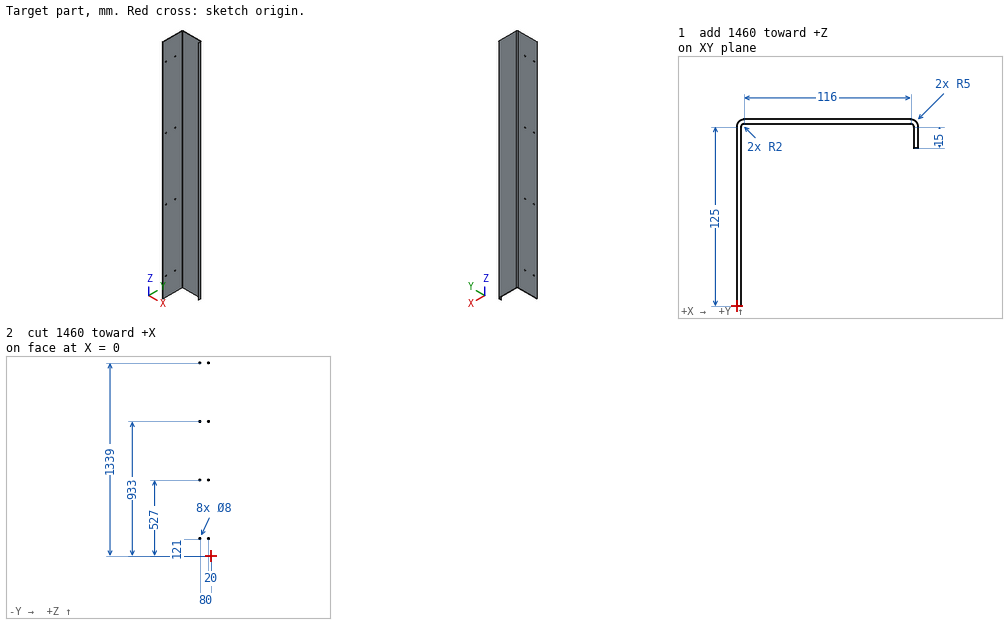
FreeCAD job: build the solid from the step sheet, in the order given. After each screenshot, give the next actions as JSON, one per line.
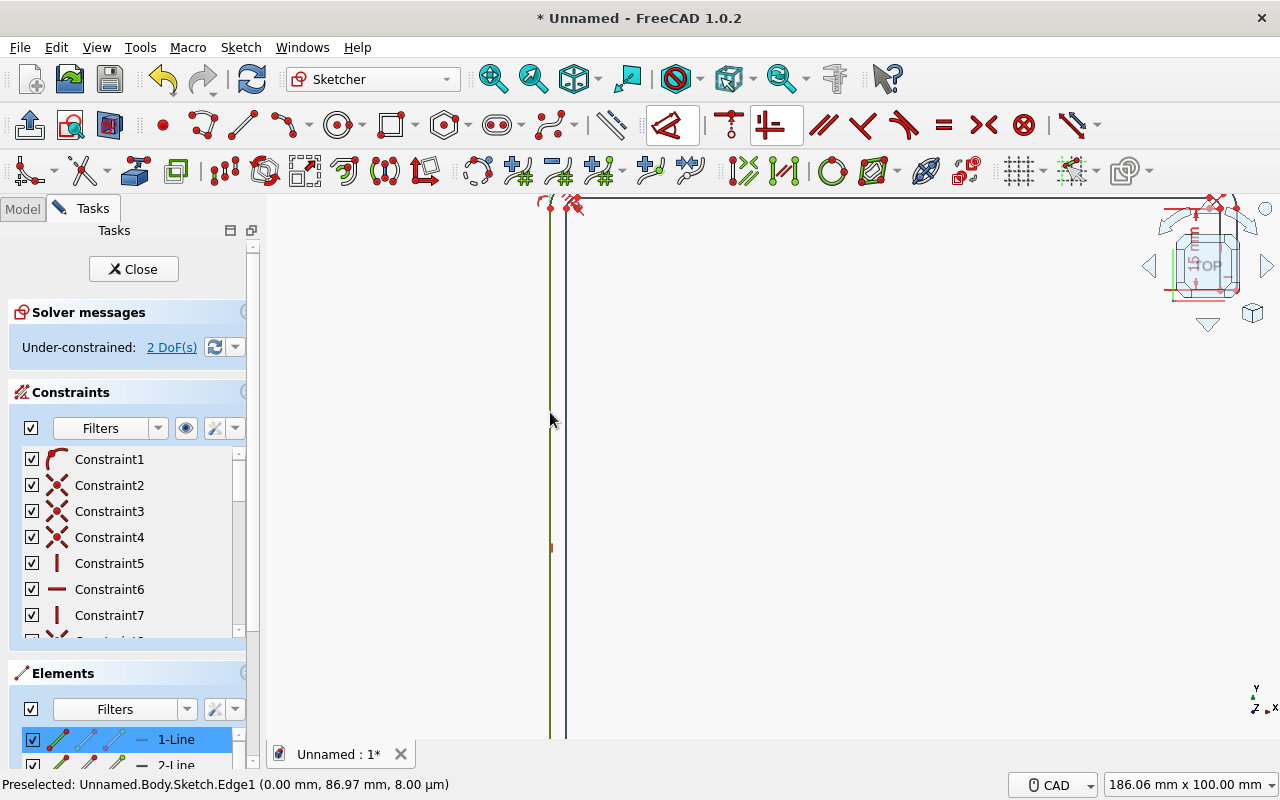
{"action": "left_click", "coordinate": [694, 126]}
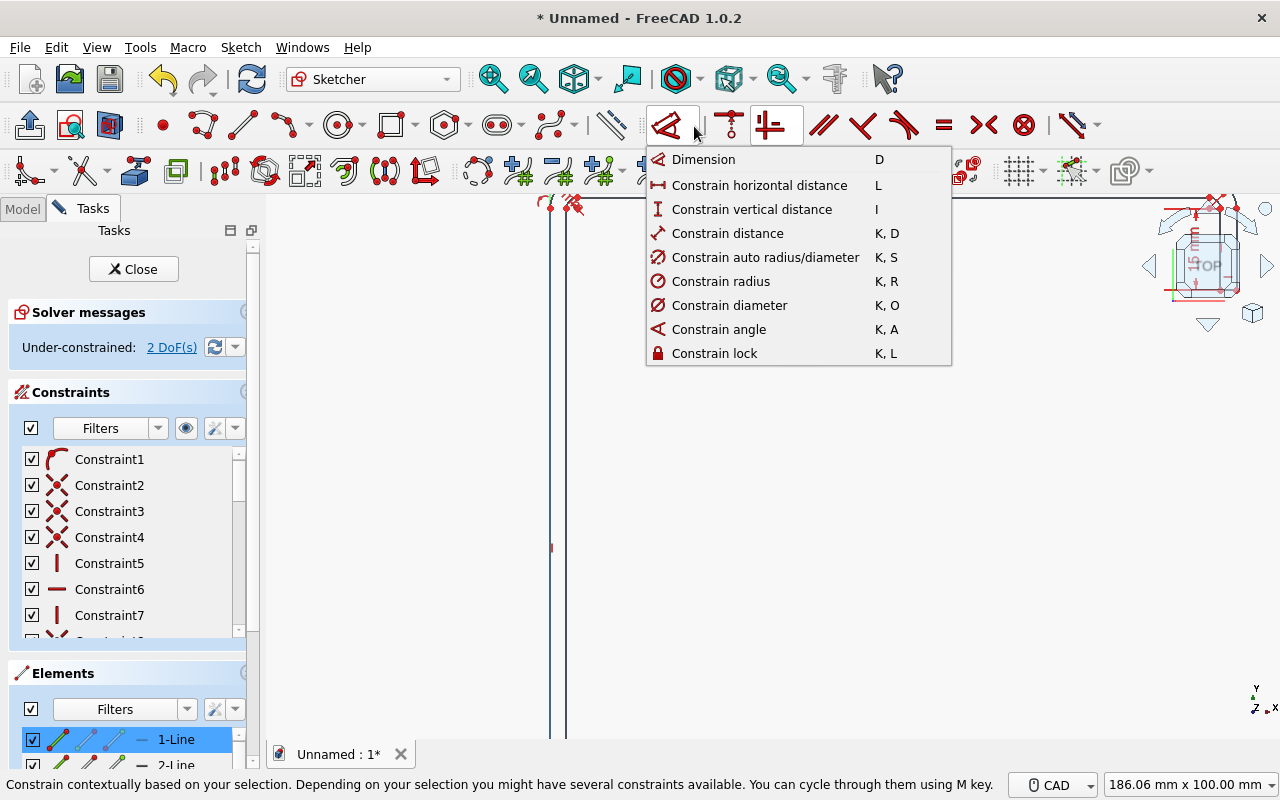
{"action": "left_click", "coordinate": [799, 209]}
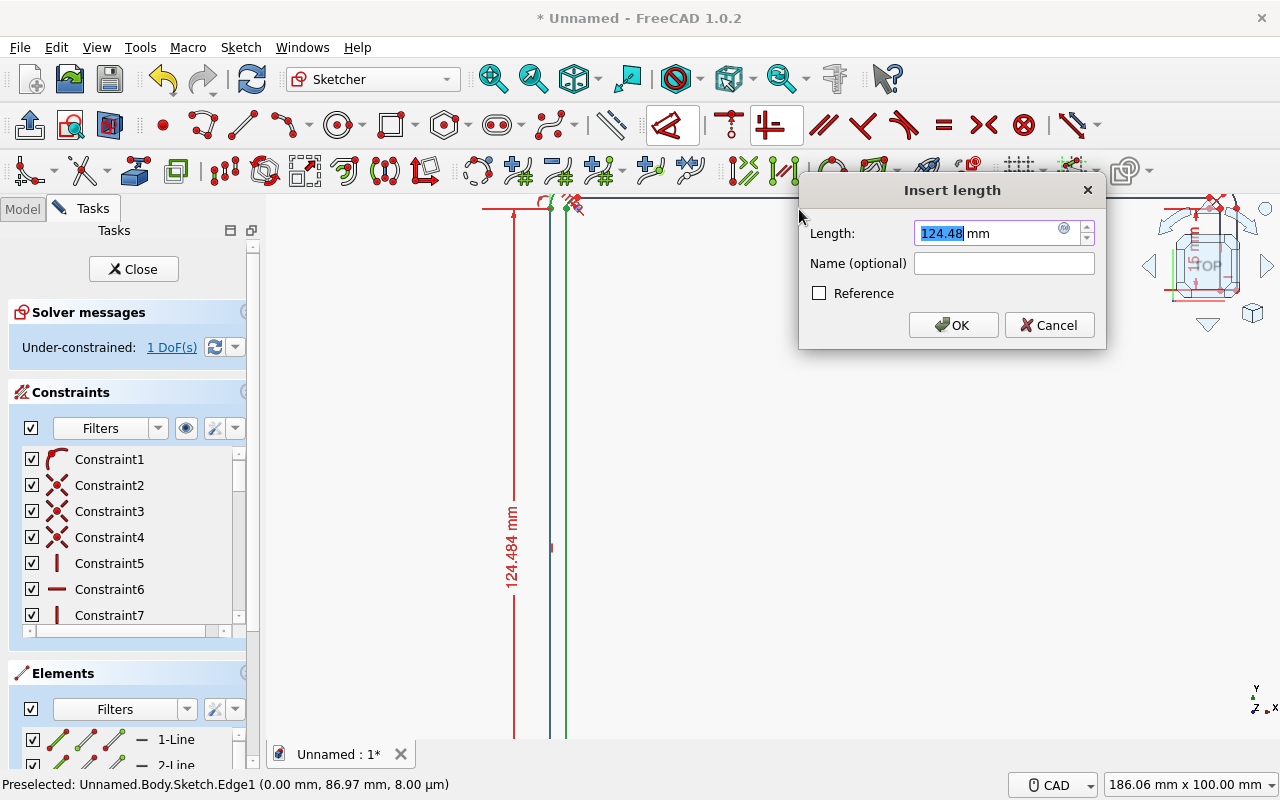
{"action": "type", "text": "125"}
{"action": "key", "text": "Return"}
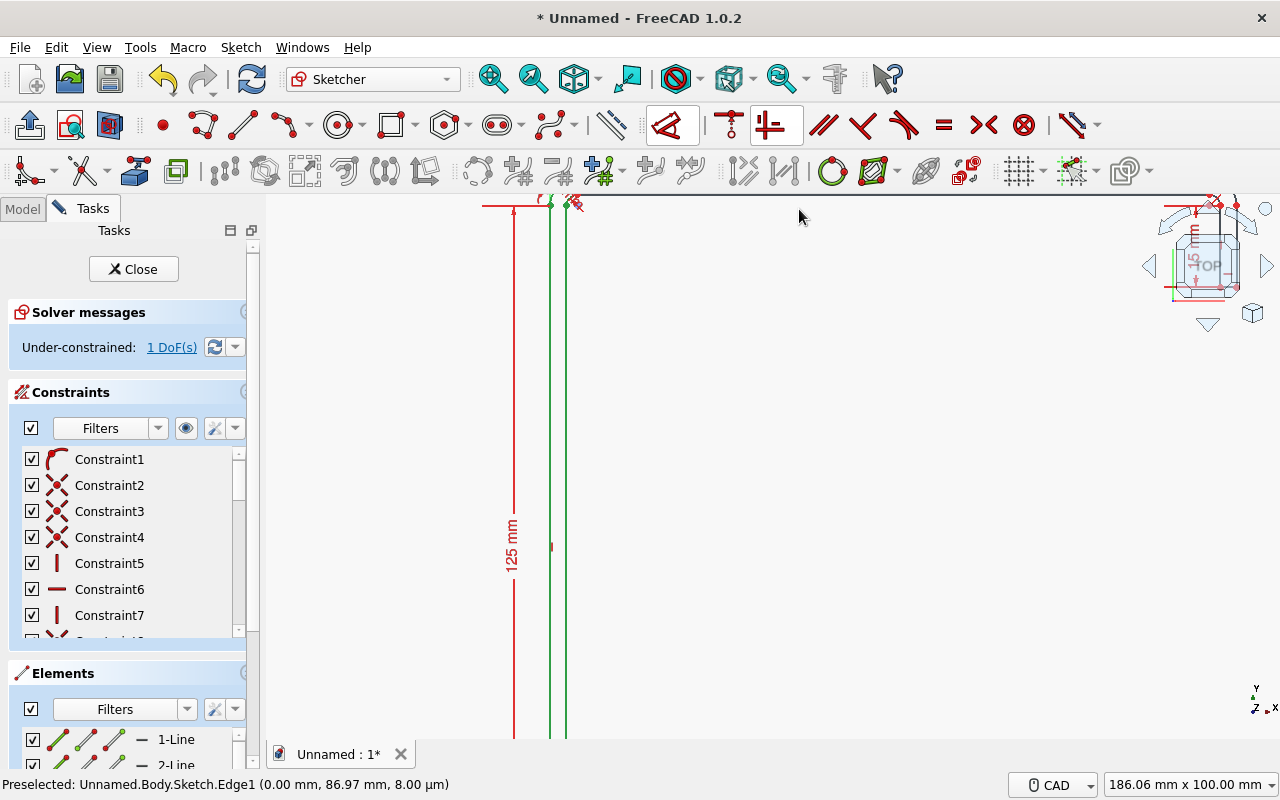
{"action": "scroll", "coordinate": [550, 412], "scroll_direction": "down", "scroll_amount": 4}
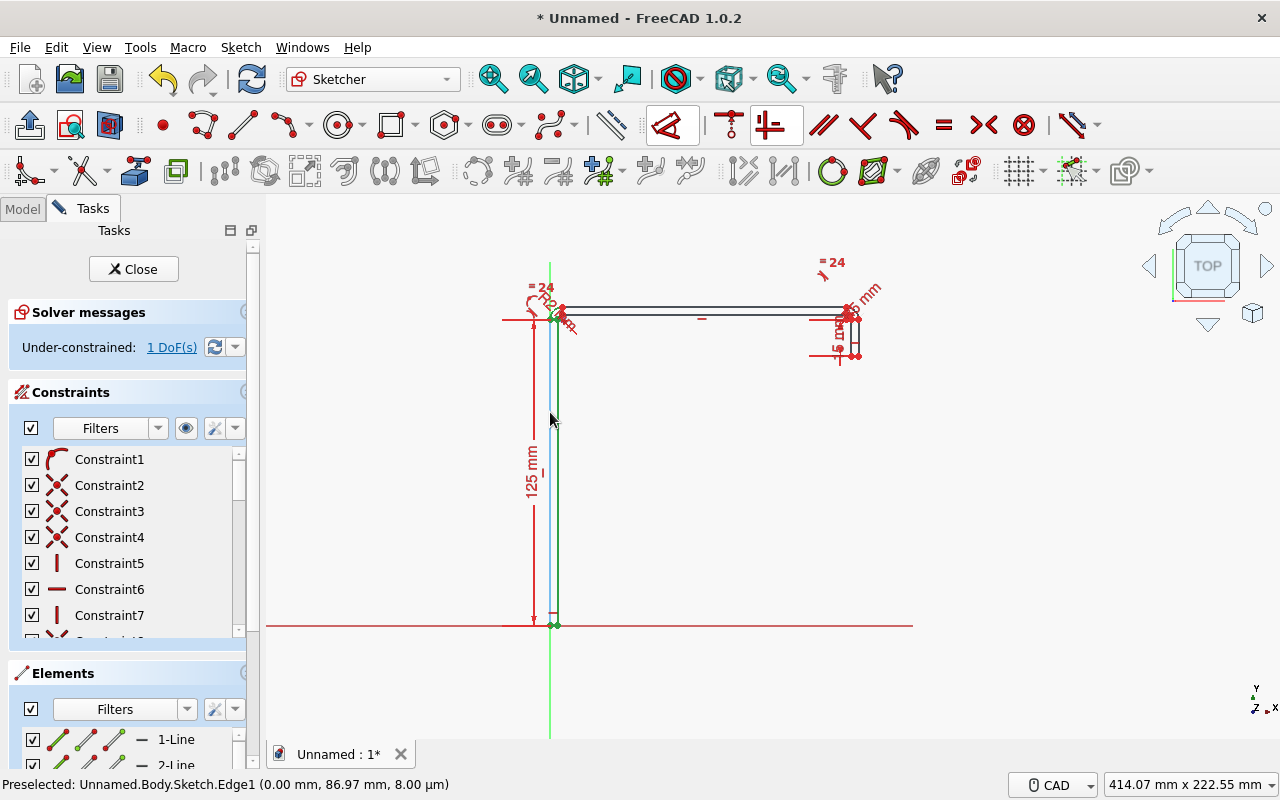
{"action": "scroll", "coordinate": [648, 315], "scroll_direction": "up", "scroll_amount": 4}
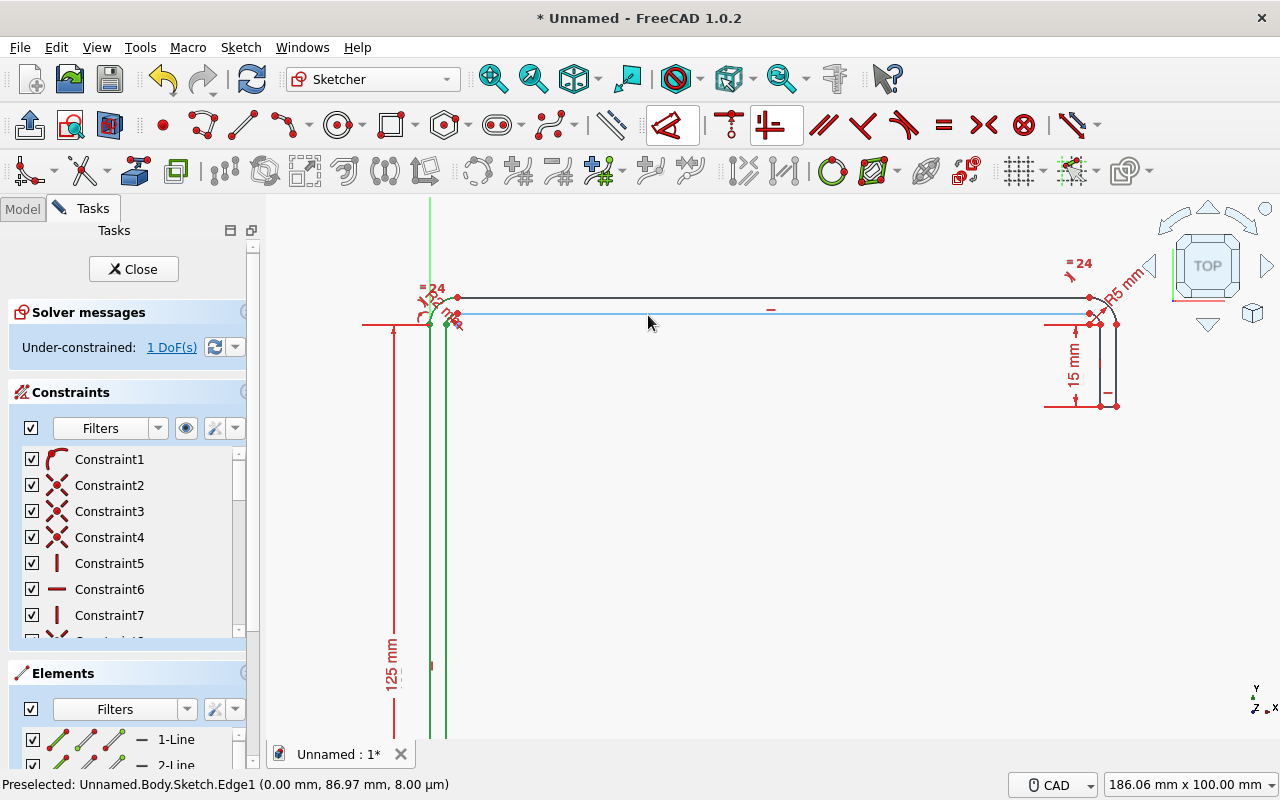
{"action": "left_click", "coordinate": [647, 314]}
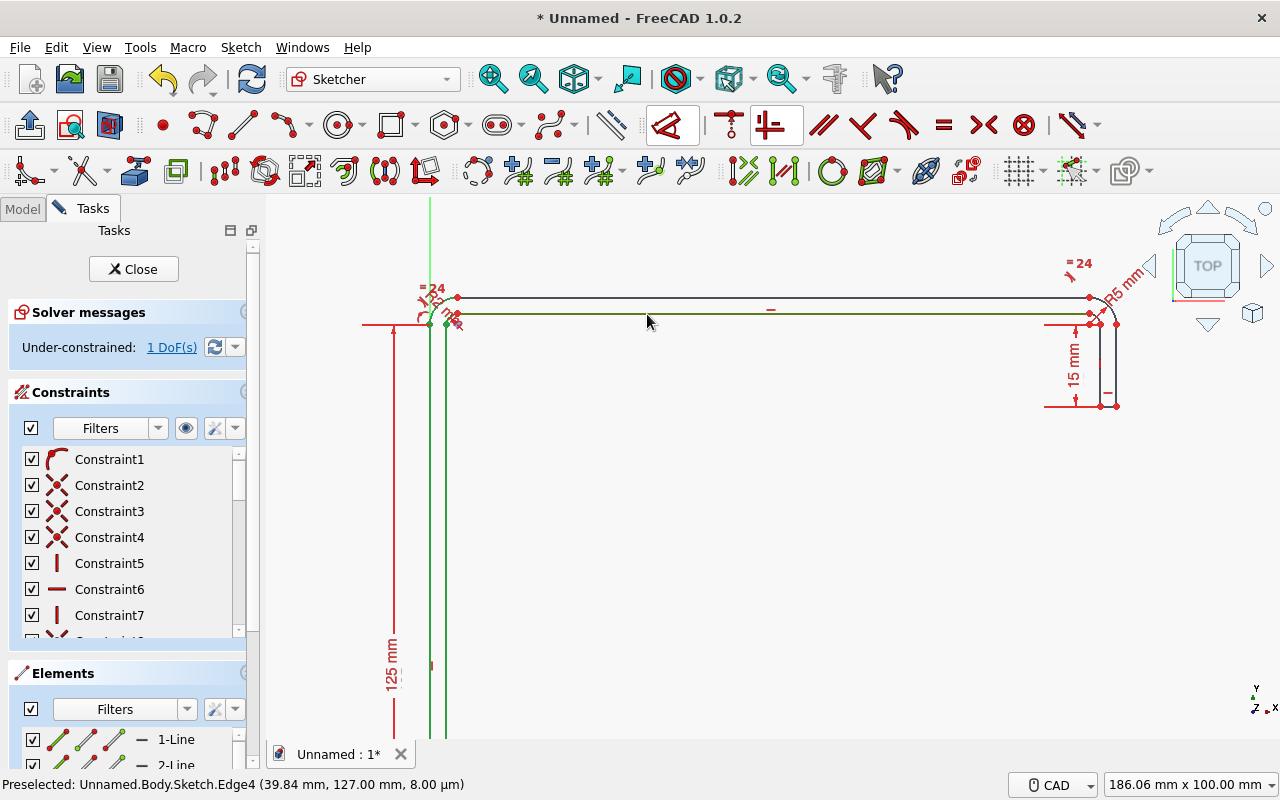
{"action": "key", "text": "l"}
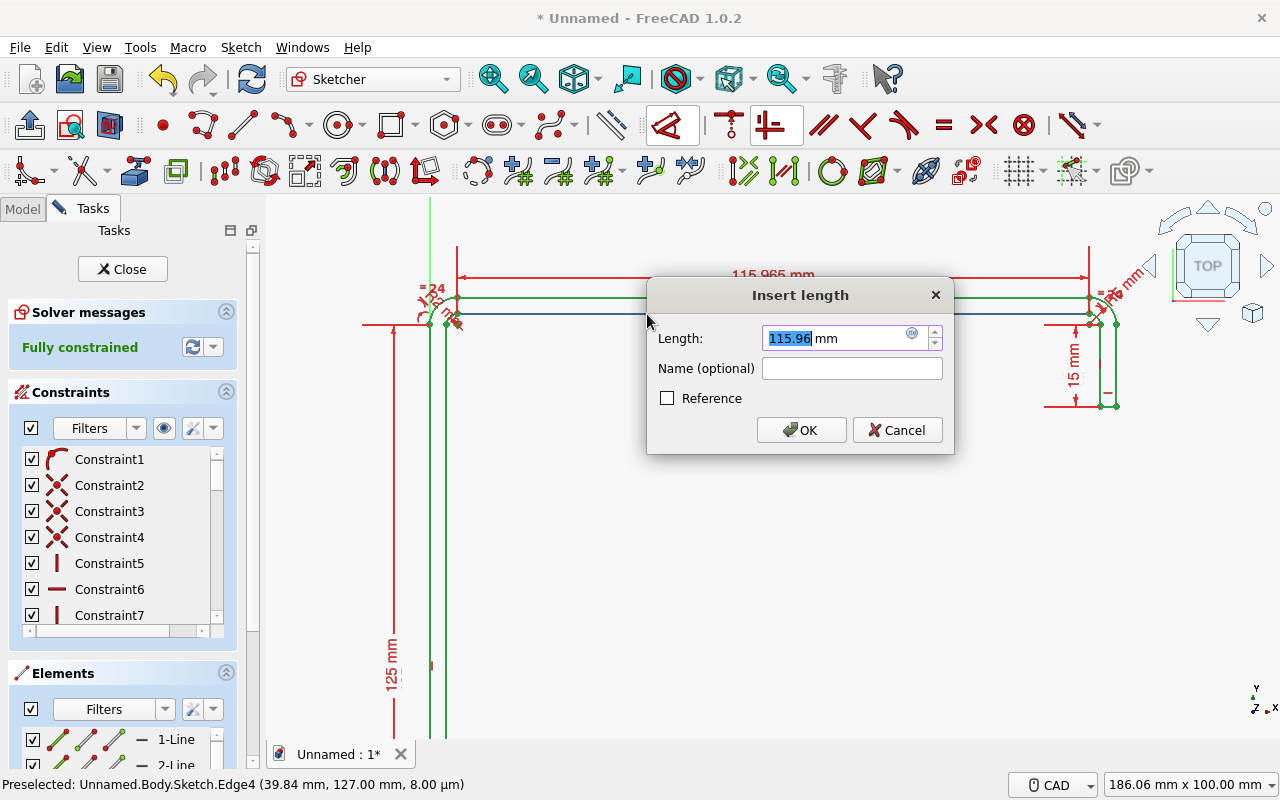
{"action": "type", "text": "116"}
{"action": "key", "text": "Return"}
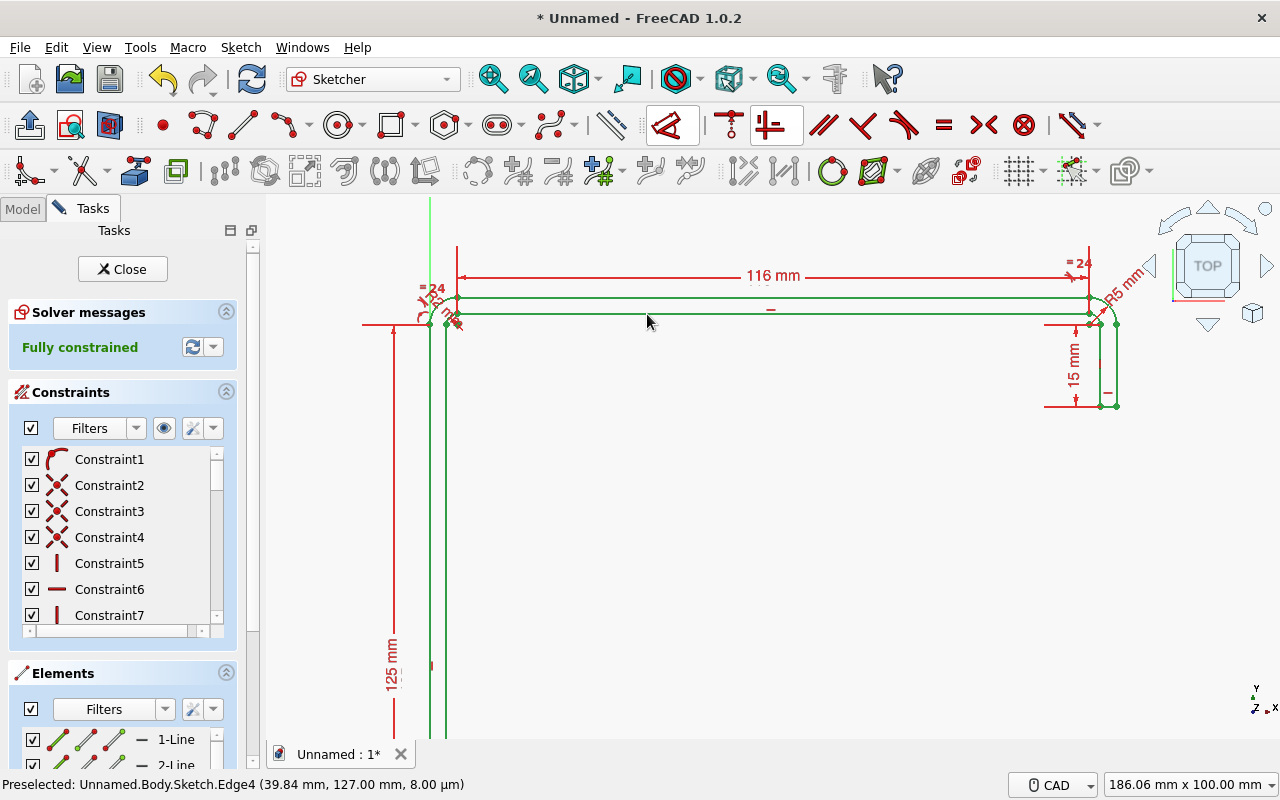
{"action": "left_click", "coordinate": [123, 269]}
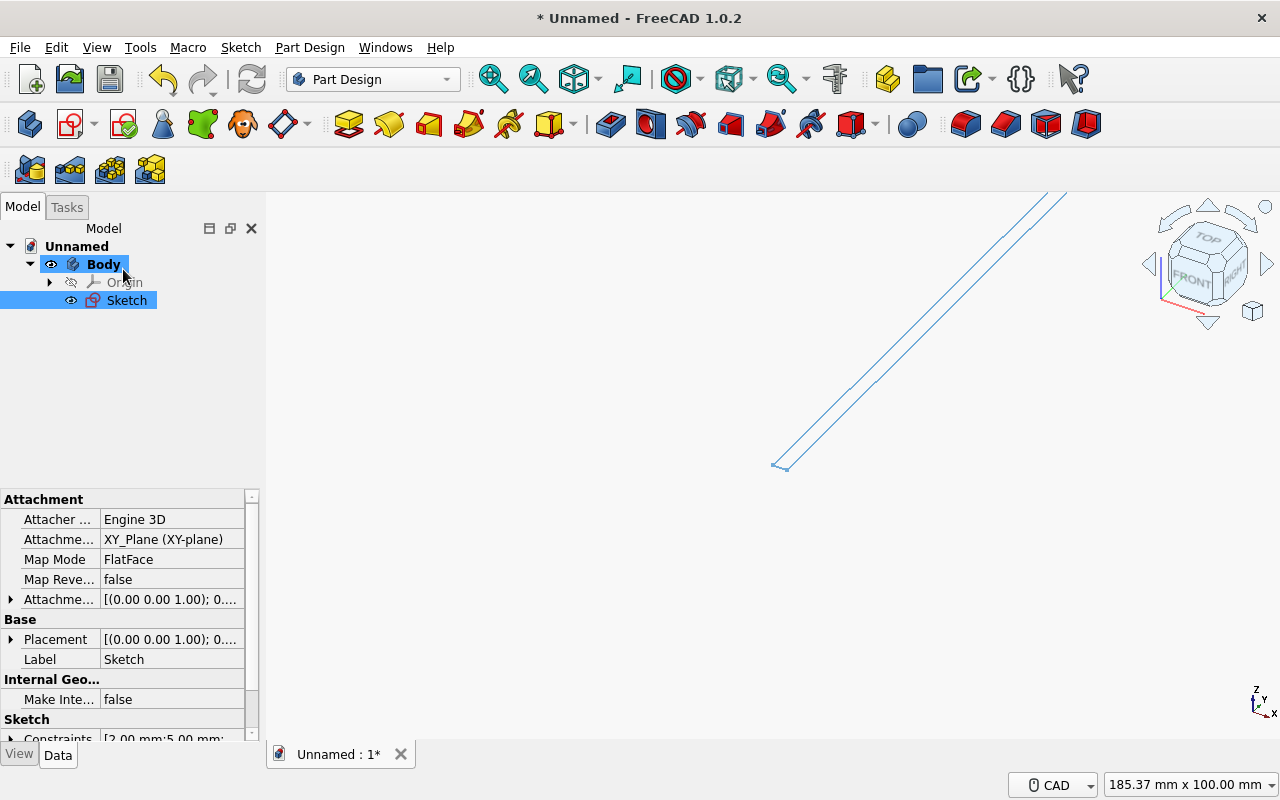
{"action": "left_click", "coordinate": [350, 124]}